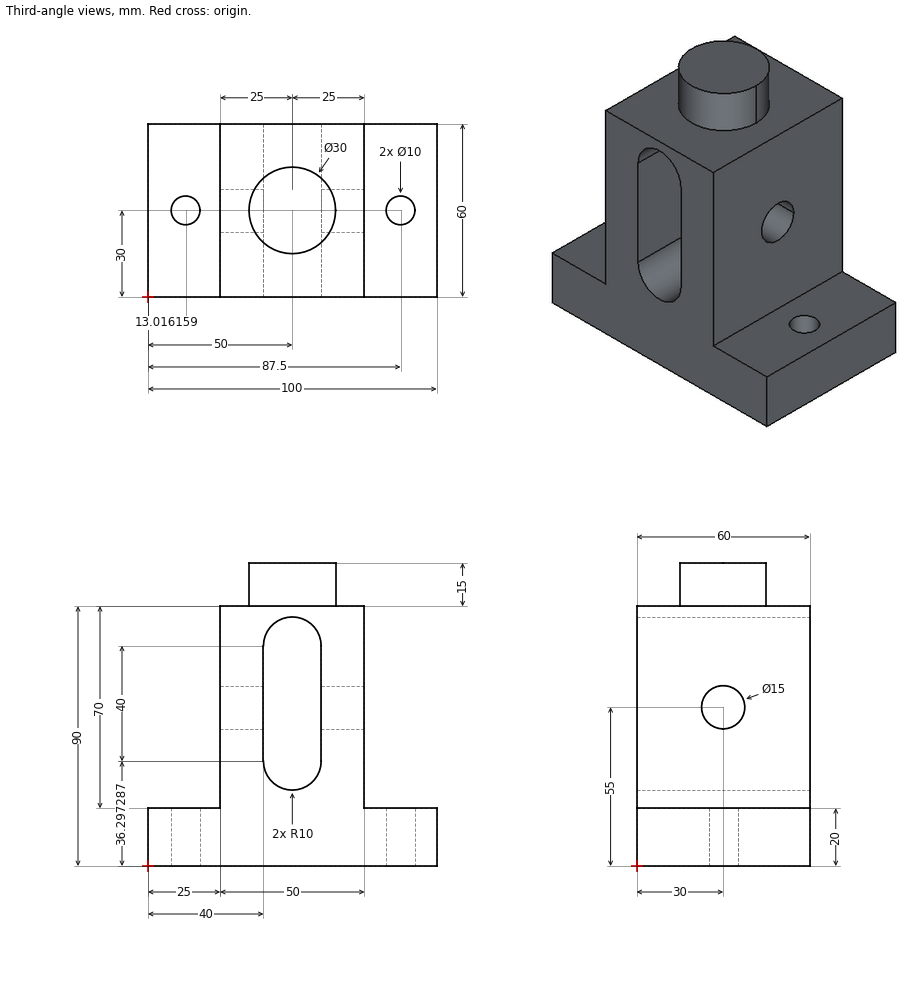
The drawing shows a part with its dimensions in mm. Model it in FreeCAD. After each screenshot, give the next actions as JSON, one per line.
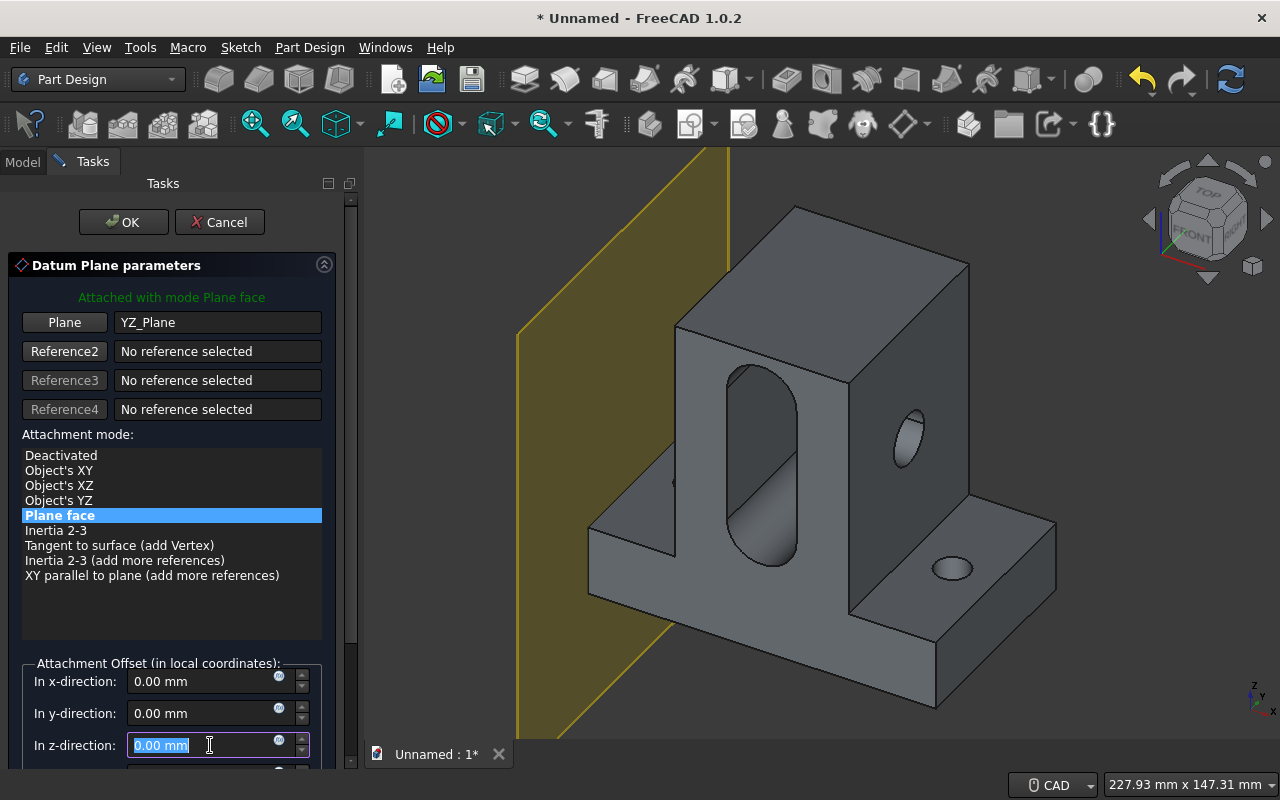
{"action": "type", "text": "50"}
{"action": "key", "text": "Tab"}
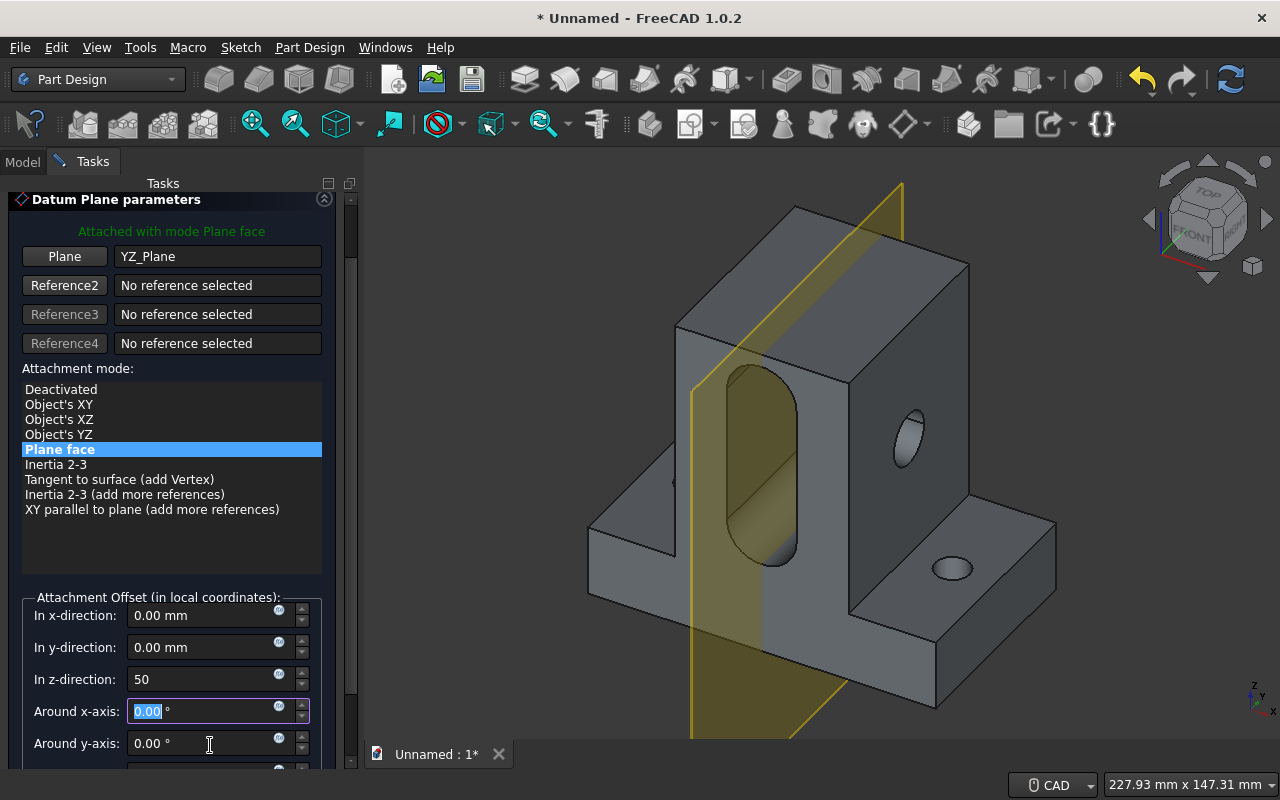
{"action": "scroll", "coordinate": [351, 480], "scroll_direction": "up", "scroll_amount": 2}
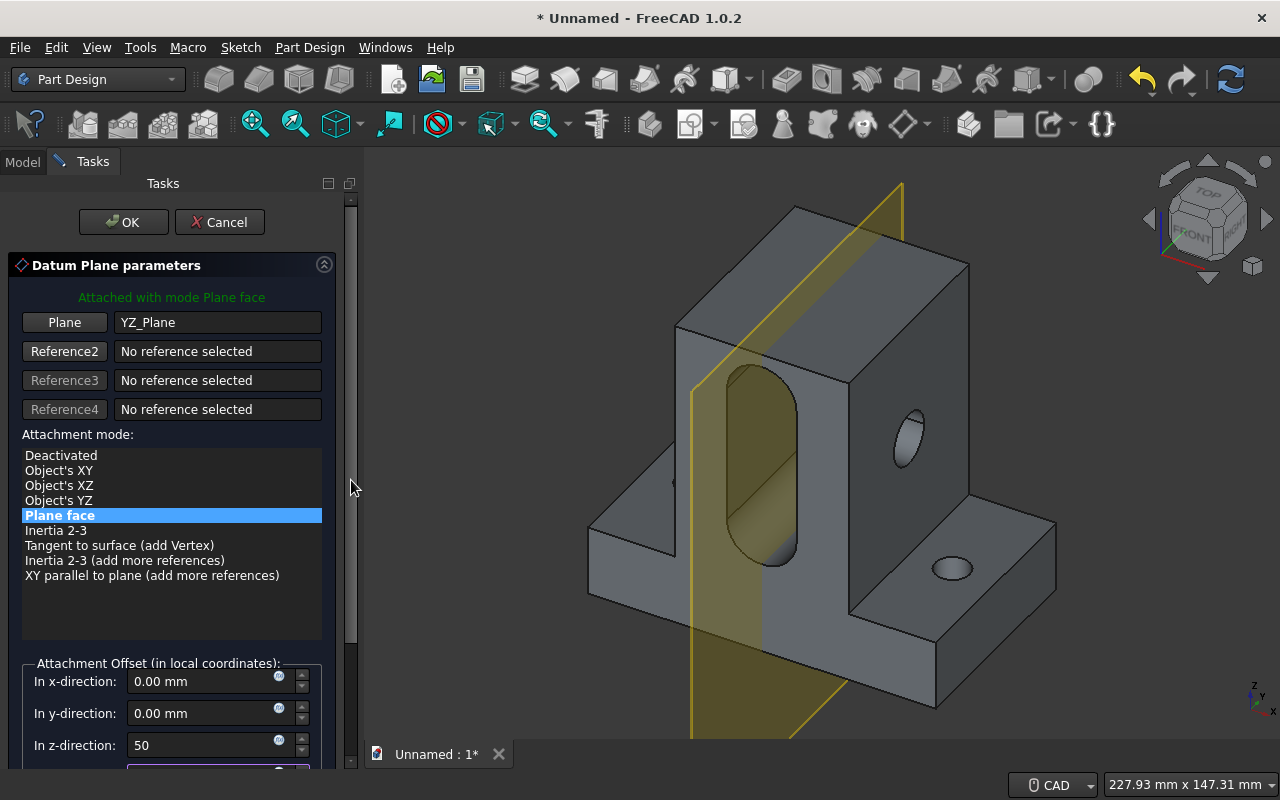
{"action": "left_click", "coordinate": [124, 222]}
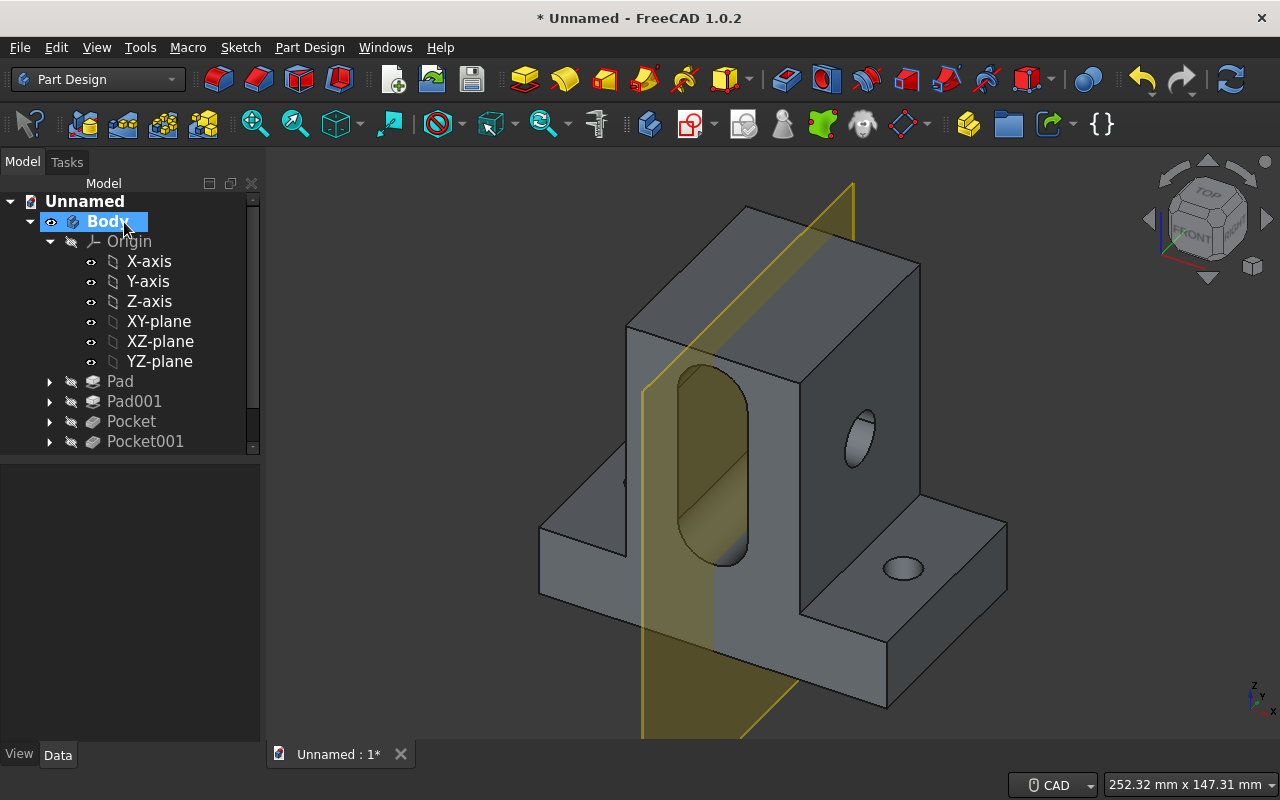
{"action": "scroll", "coordinate": [100, 317], "scroll_direction": "down", "scroll_amount": 3}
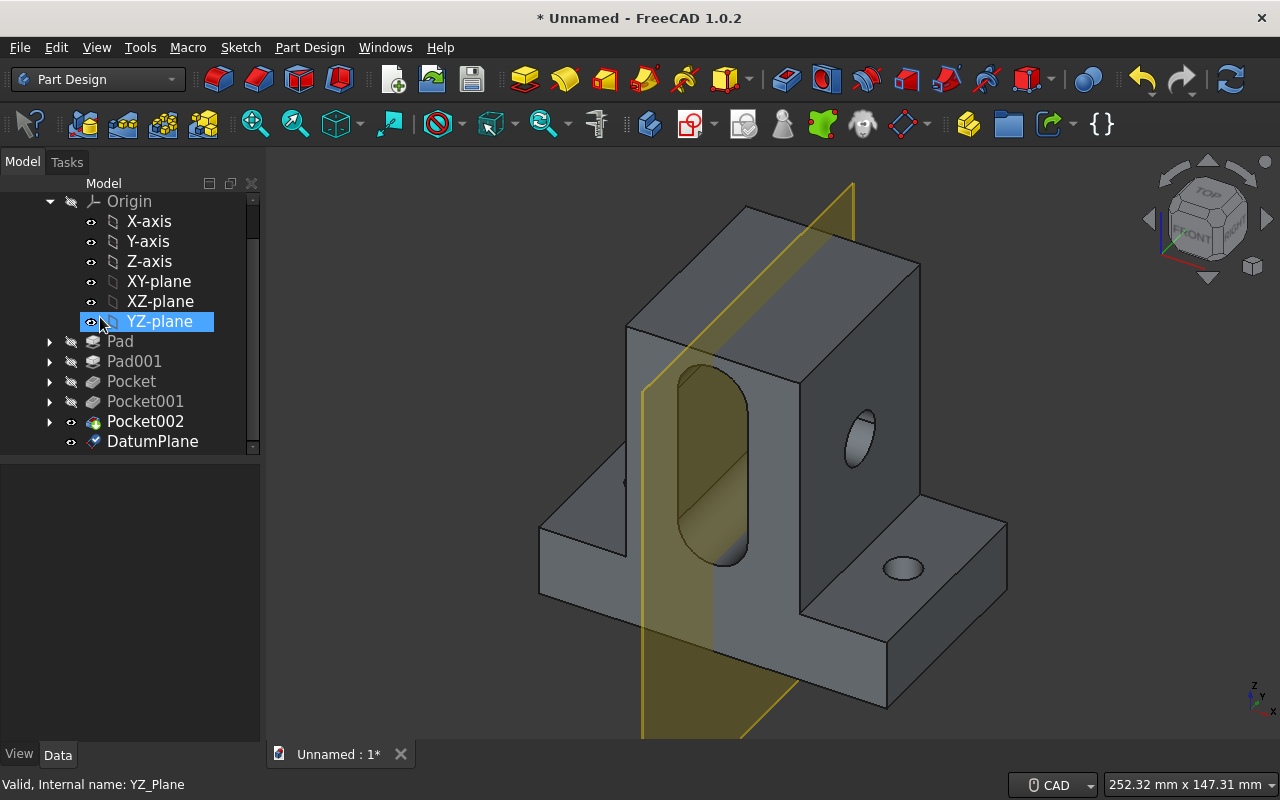
{"action": "left_click", "coordinate": [116, 442]}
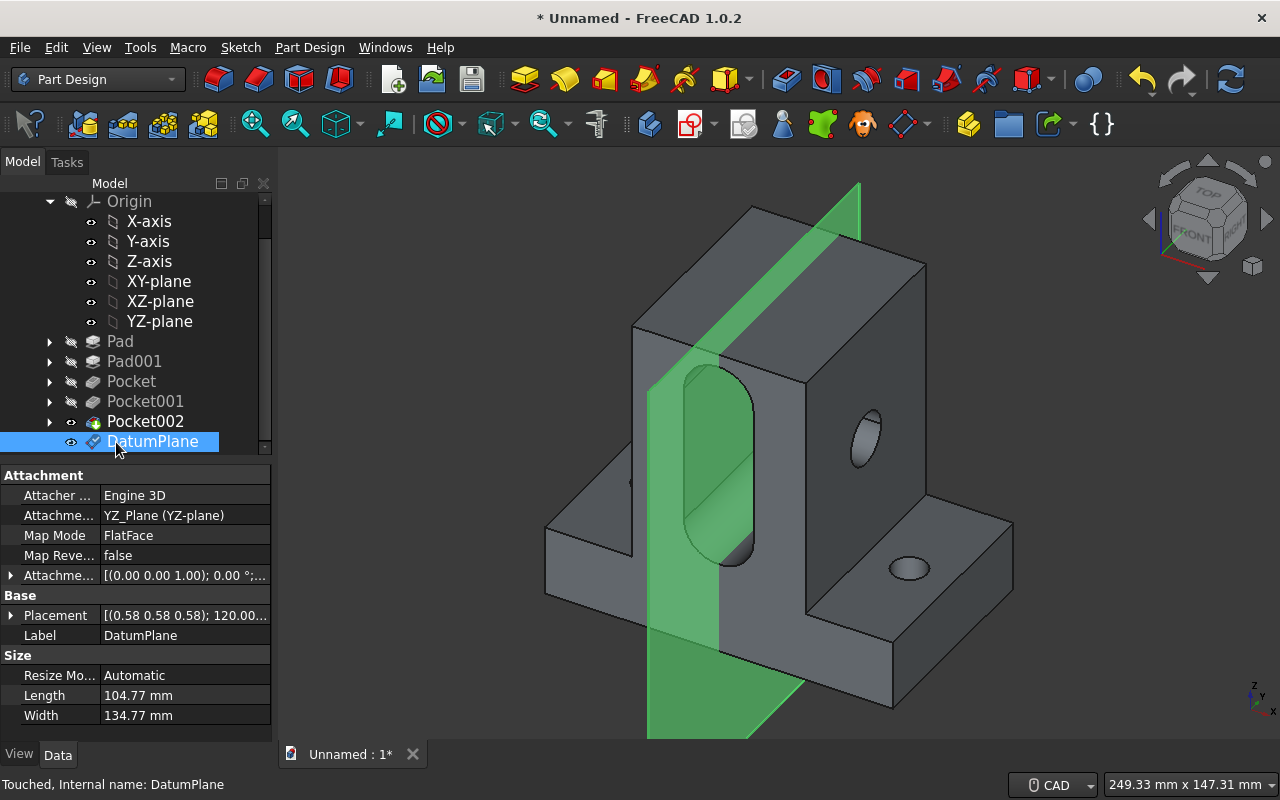
{"action": "left_click", "coordinate": [690, 124]}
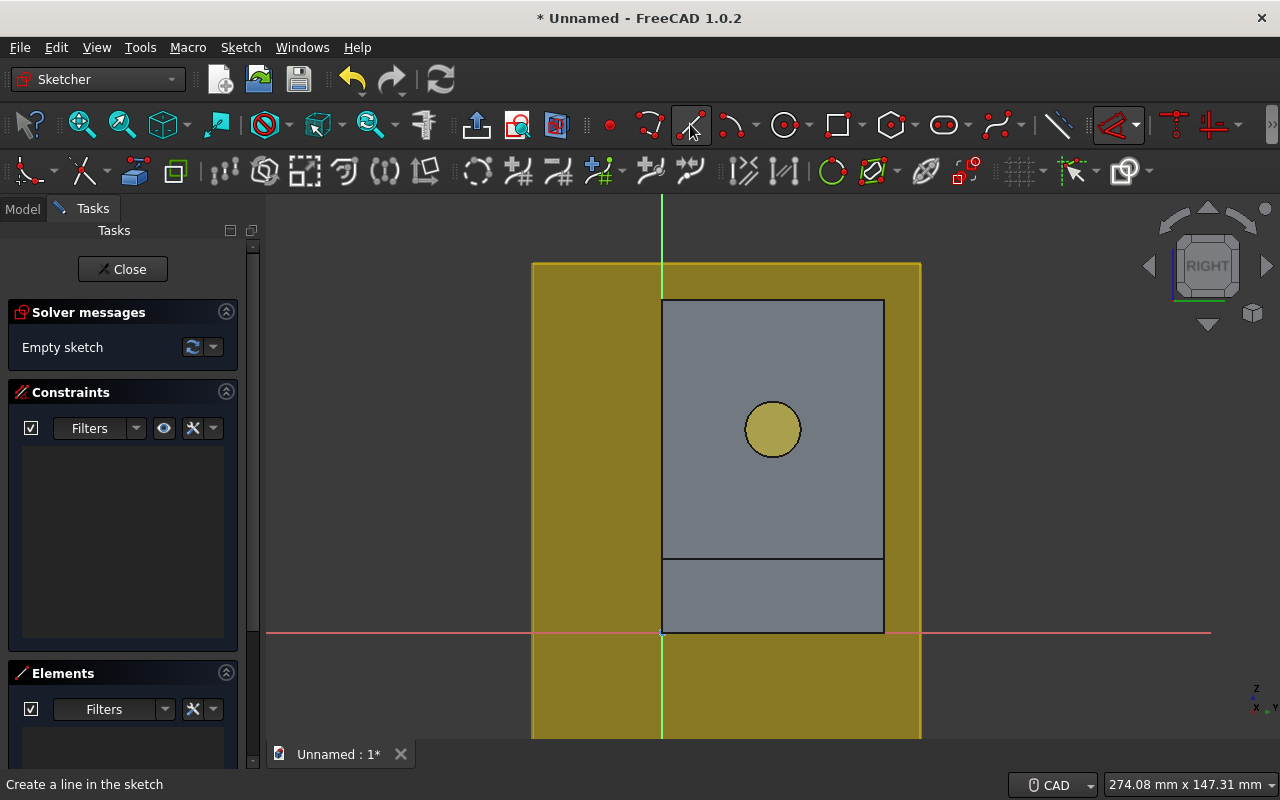
{"action": "key", "text": "q s"}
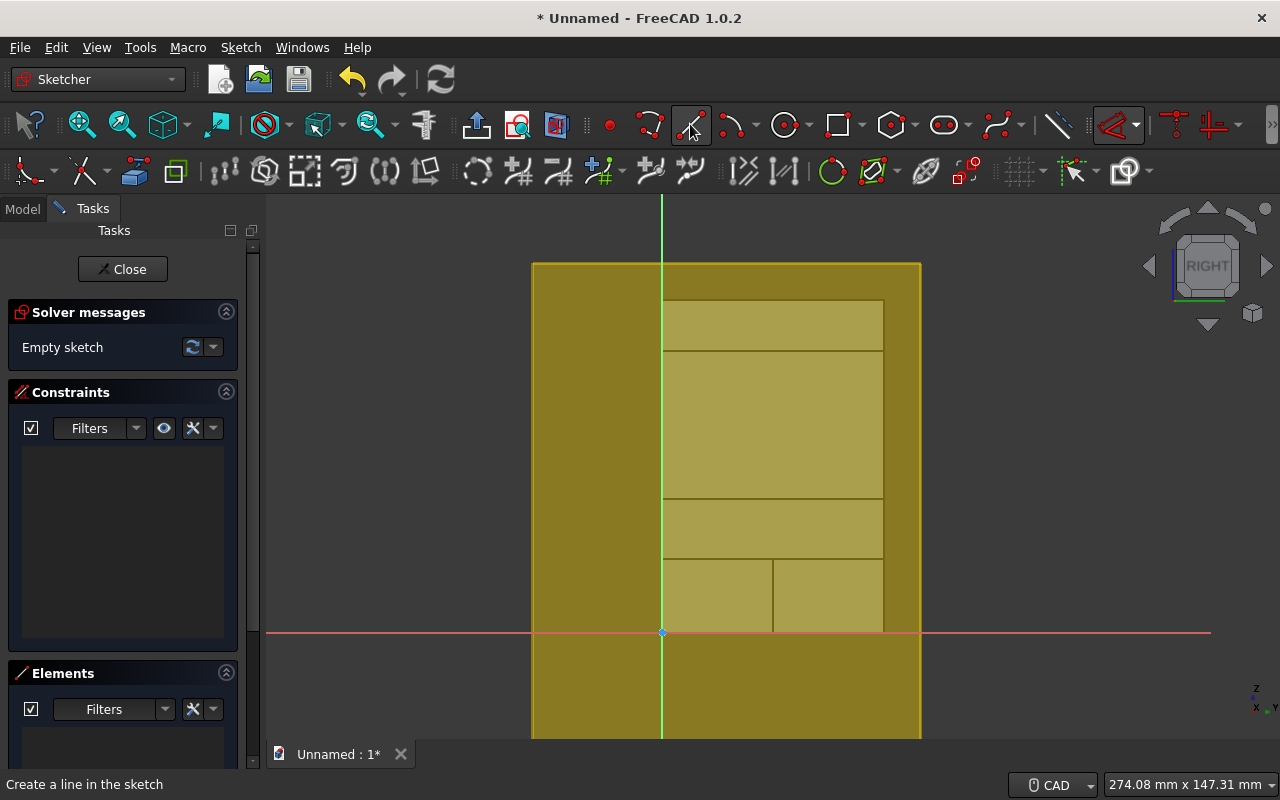
{"action": "scroll", "coordinate": [787, 422], "scroll_direction": "up", "scroll_amount": 9}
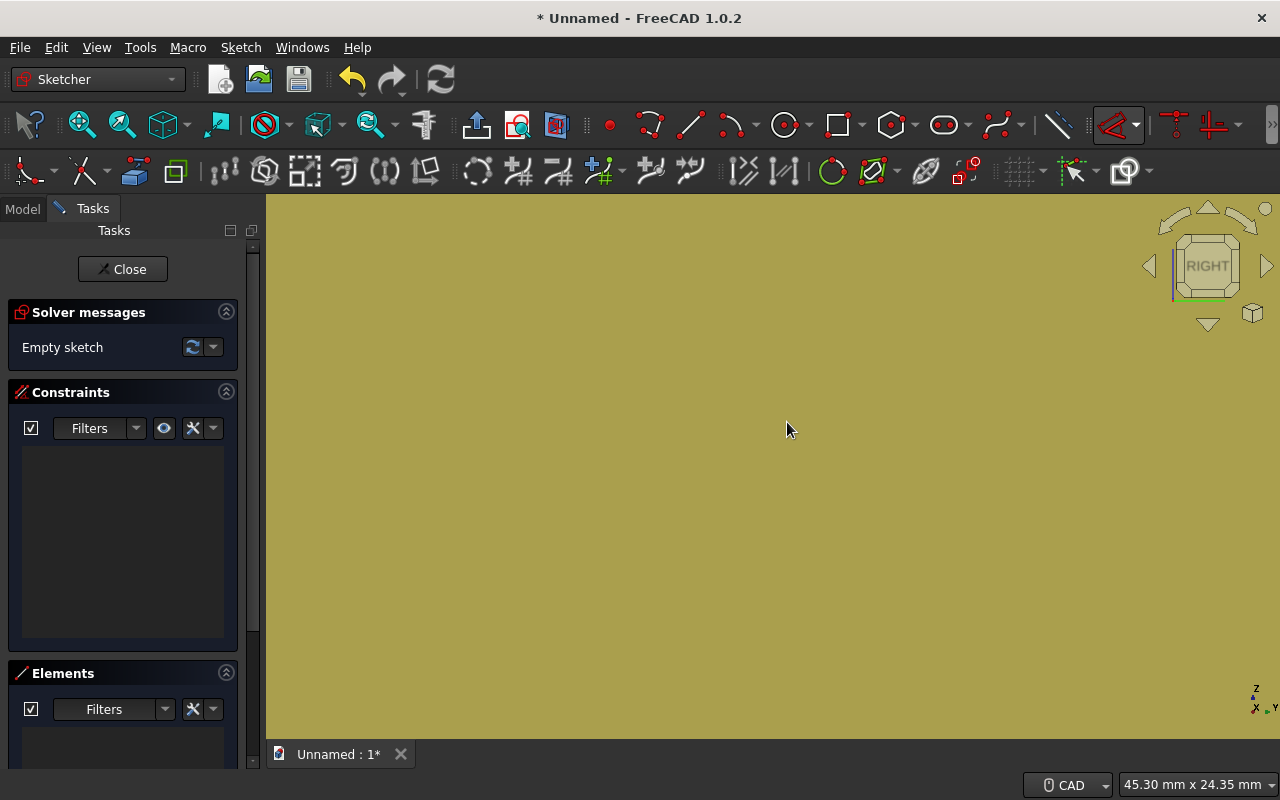
{"action": "left_click", "coordinate": [786, 126]}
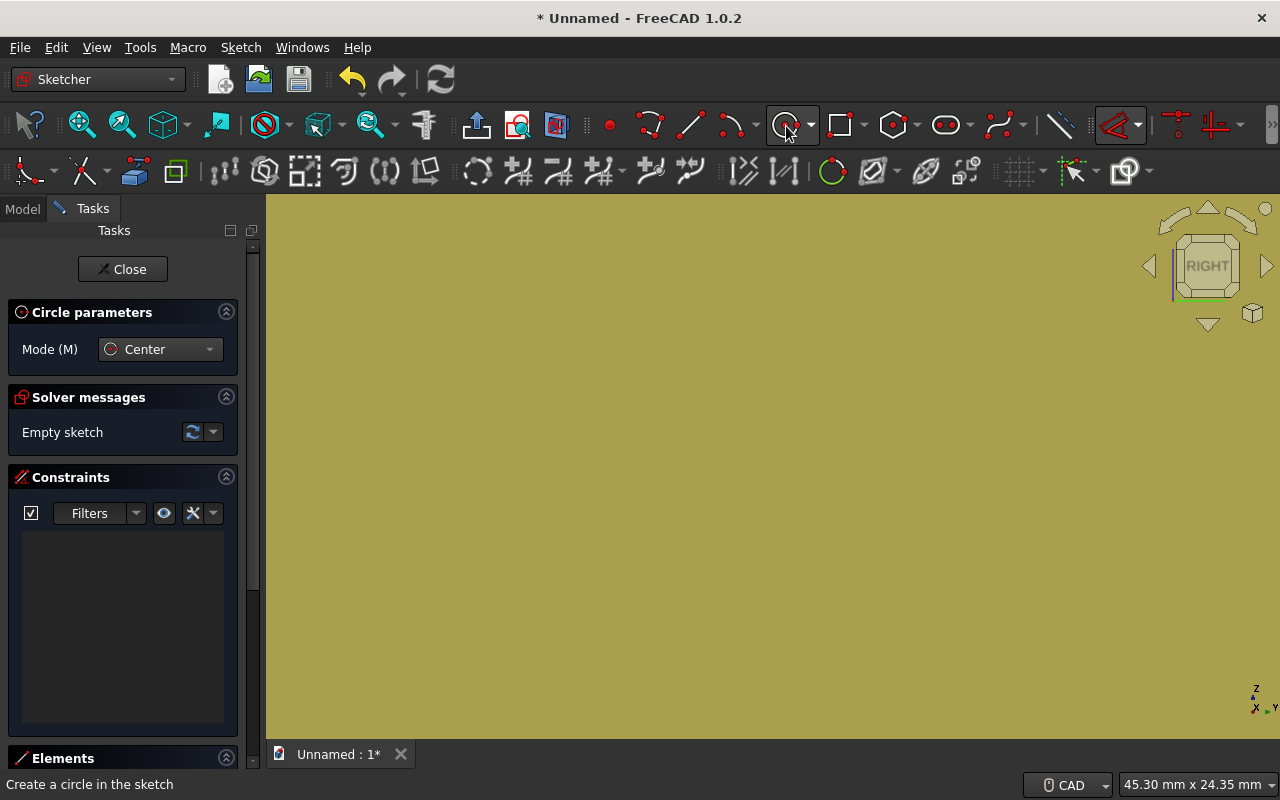
{"action": "left_click", "coordinate": [700, 465]}
{"action": "left_click", "coordinate": [818, 347]}
{"action": "key", "text": "Escape"}